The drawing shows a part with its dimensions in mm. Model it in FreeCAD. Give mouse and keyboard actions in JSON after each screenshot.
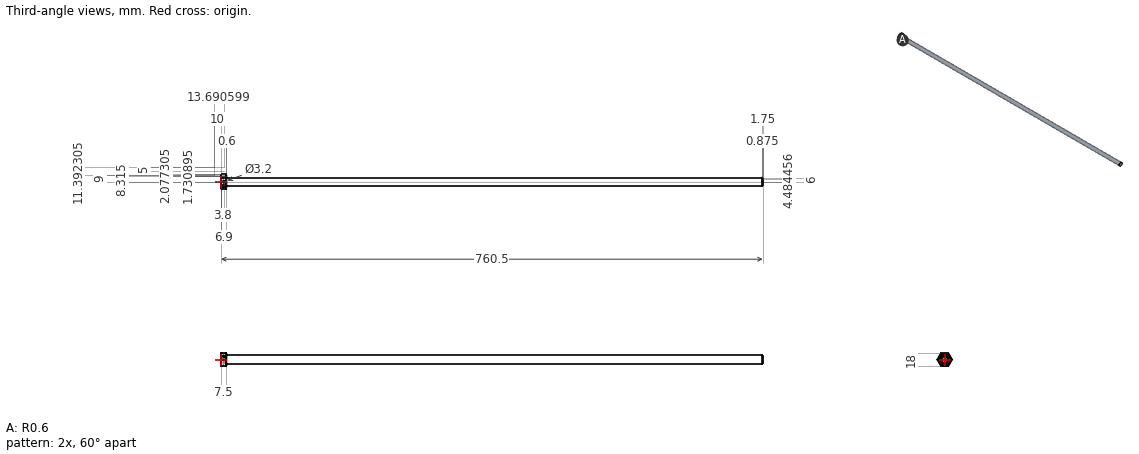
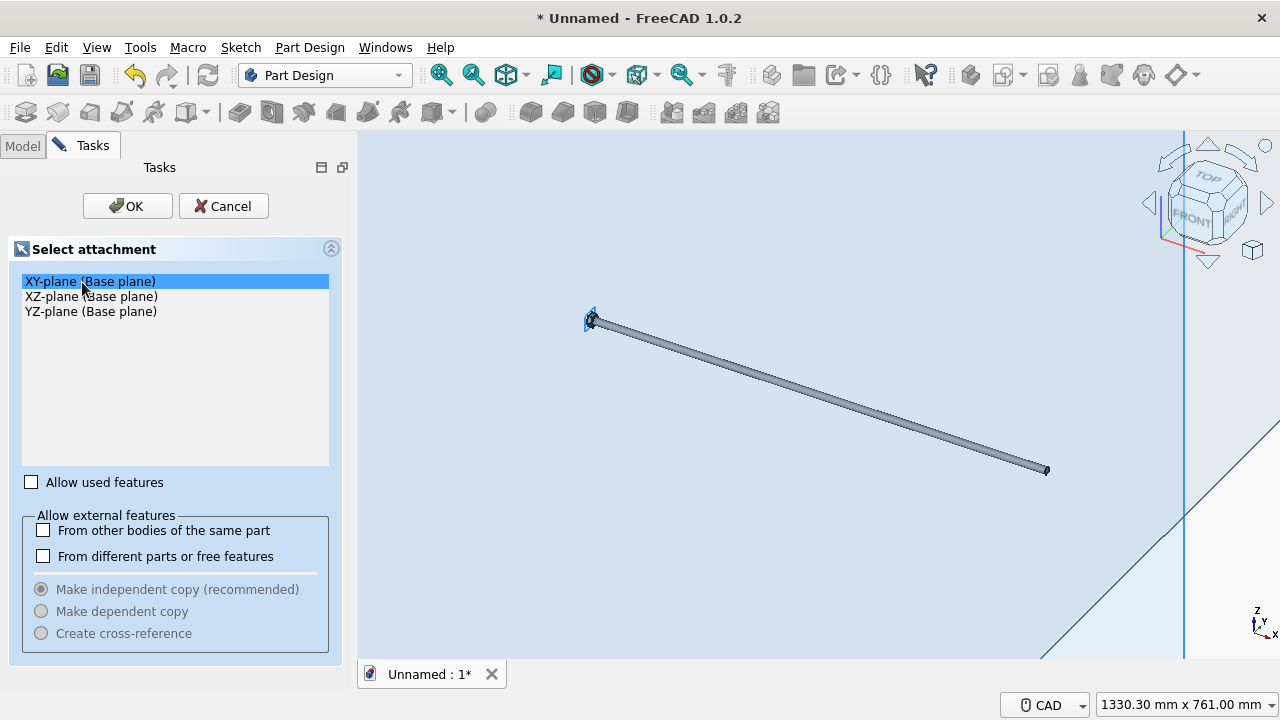
{"action": "left_click", "coordinate": [128, 206]}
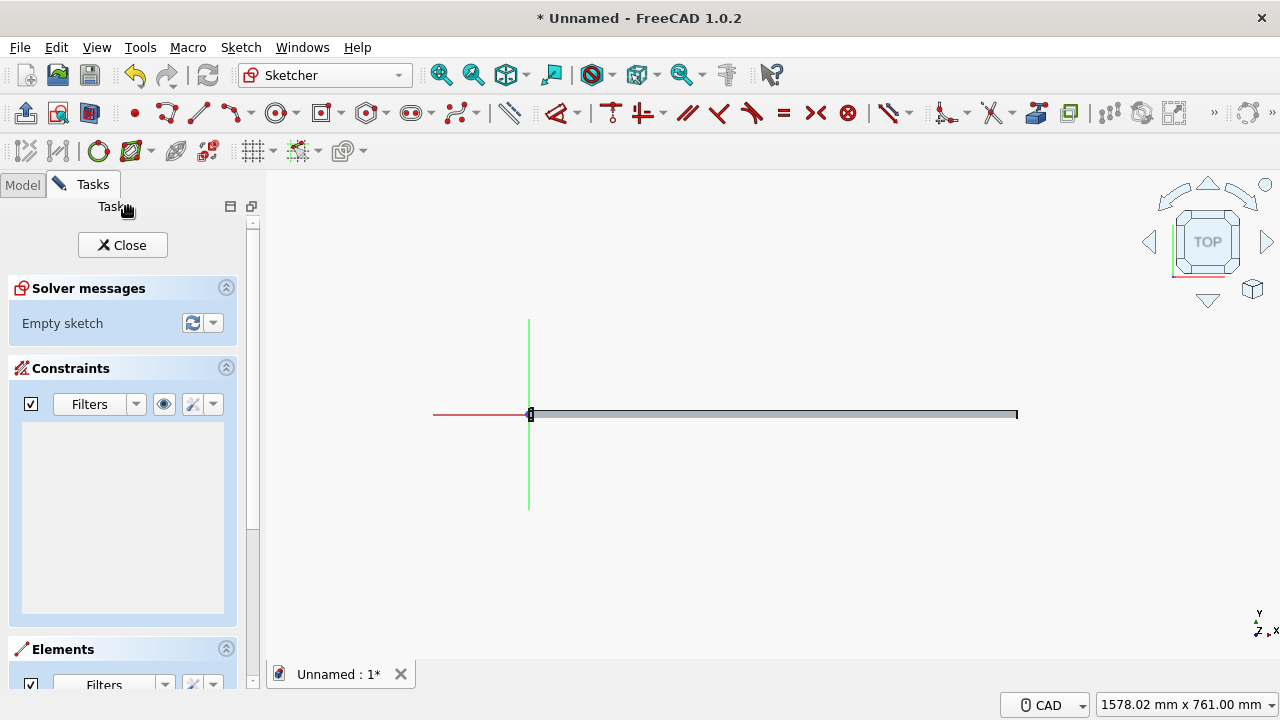
{"action": "key", "text": "q s"}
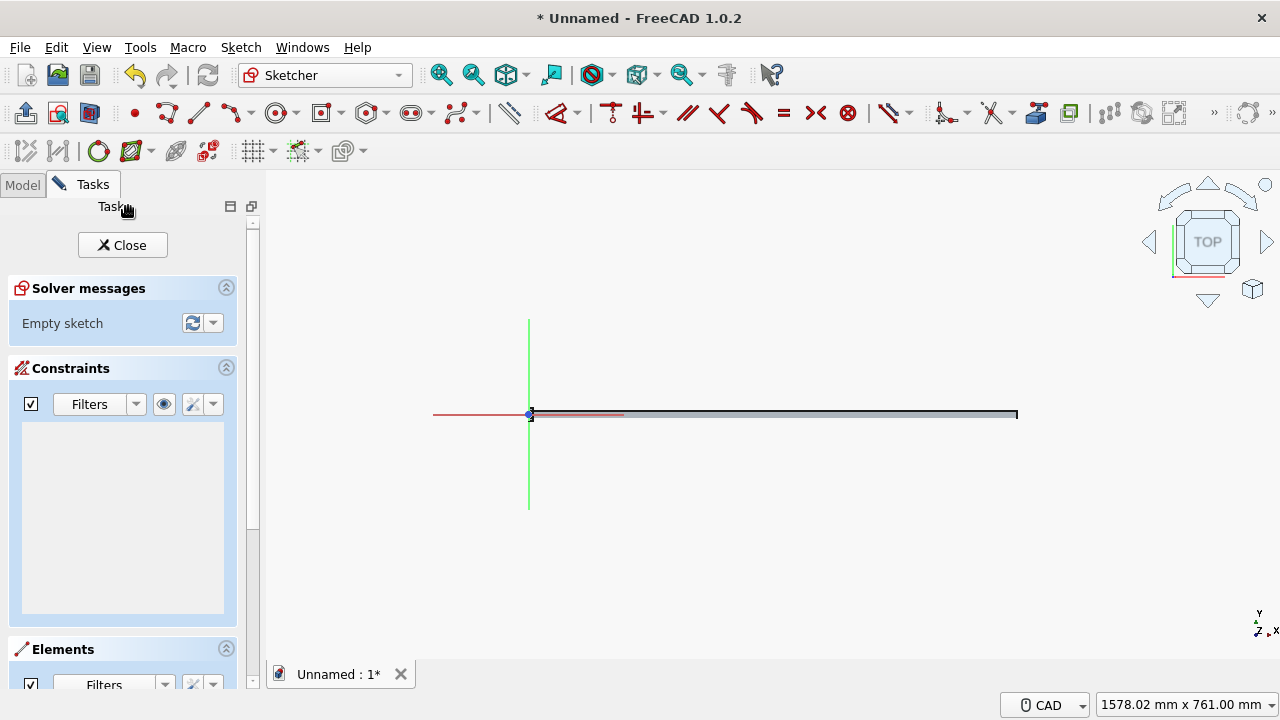
{"action": "scroll", "coordinate": [517, 408], "scroll_direction": "up", "scroll_amount": 15}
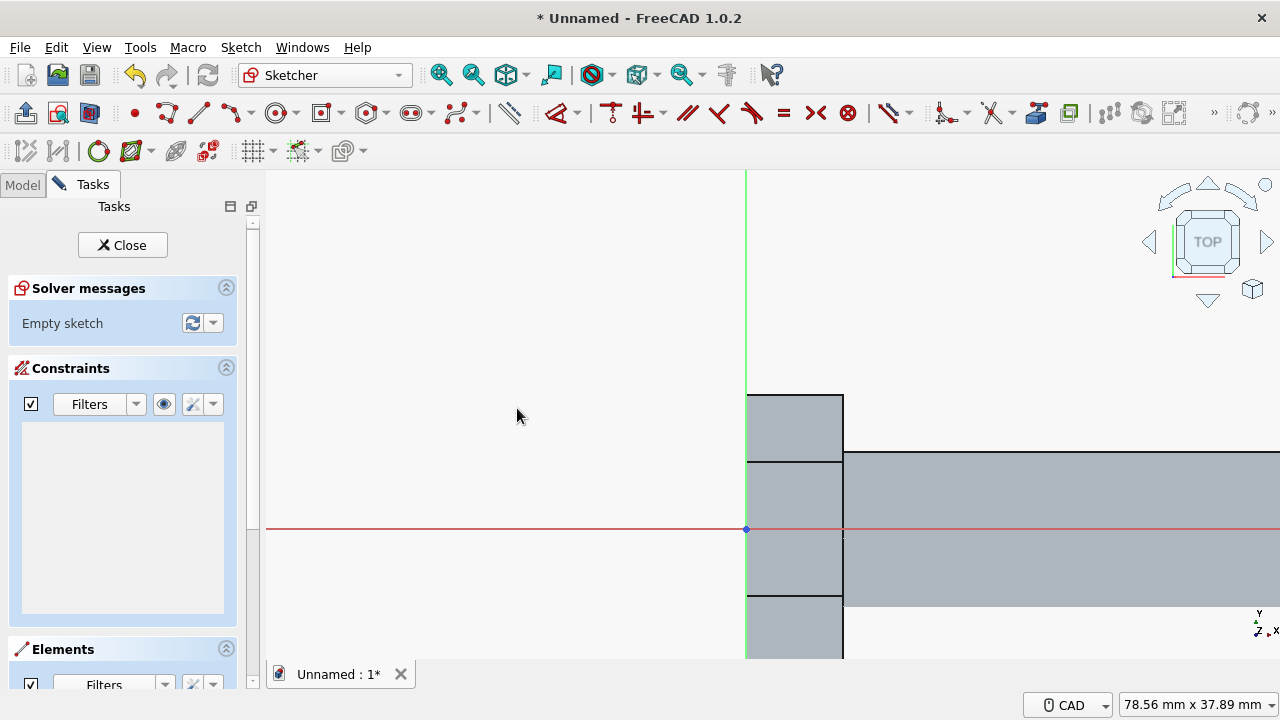
{"action": "key", "text": "g m"}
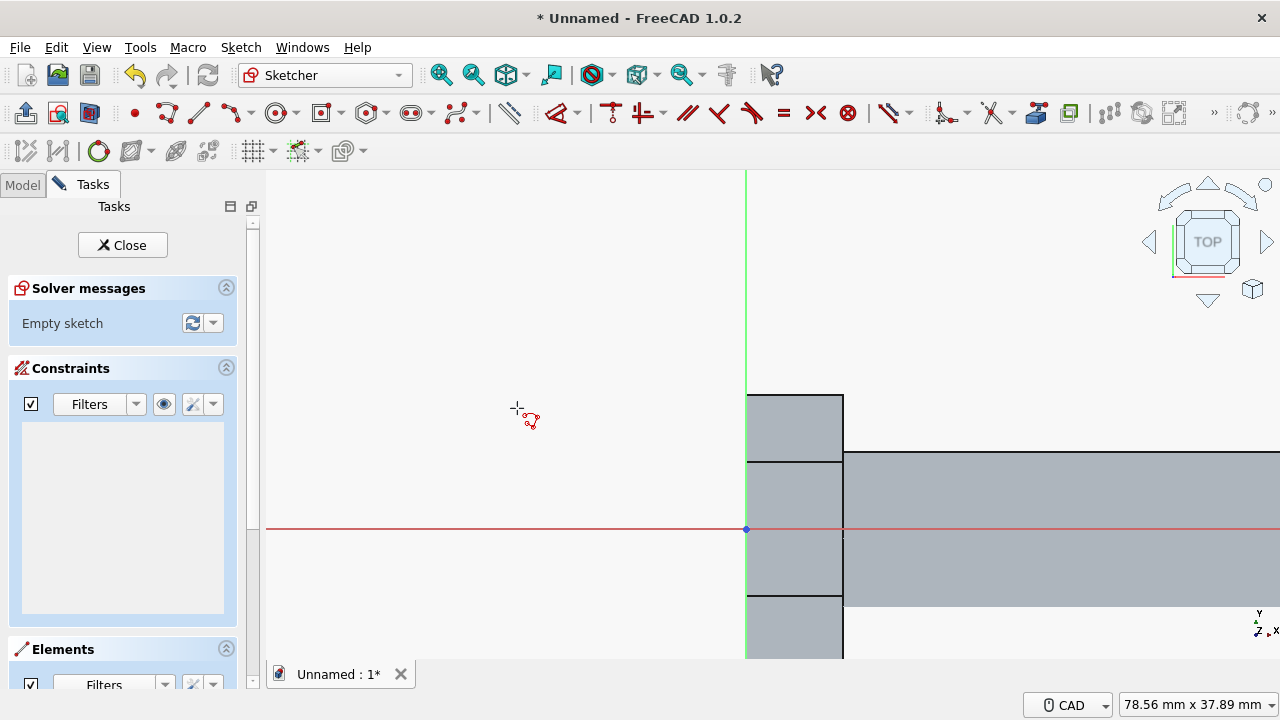
{"action": "left_click", "coordinate": [746, 413]}
{"action": "left_click", "coordinate": [794, 331]}
{"action": "left_click", "coordinate": [794, 266]}
{"action": "left_click", "coordinate": [617, 266]}
{"action": "left_click", "coordinate": [617, 413]}
{"action": "left_click", "coordinate": [746, 414]}
{"action": "key", "text": "Escape"}
{"action": "key", "text": "Escape"}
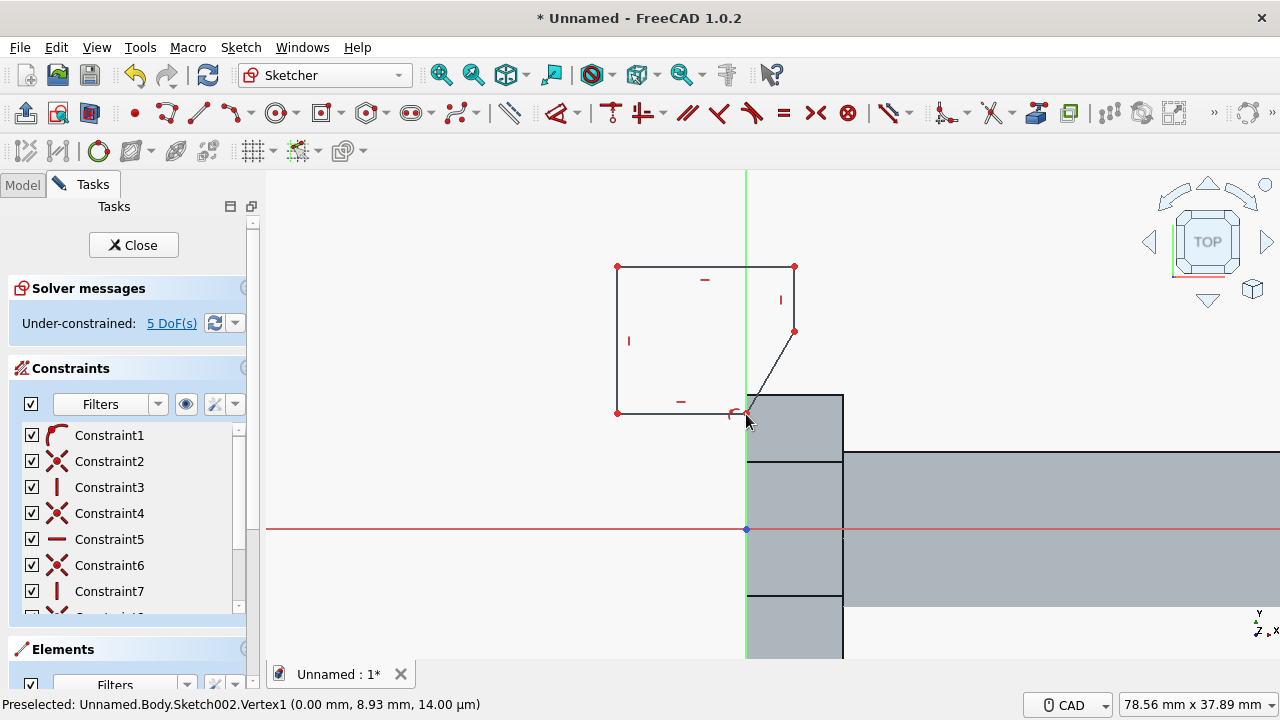
{"action": "key", "text": "d"}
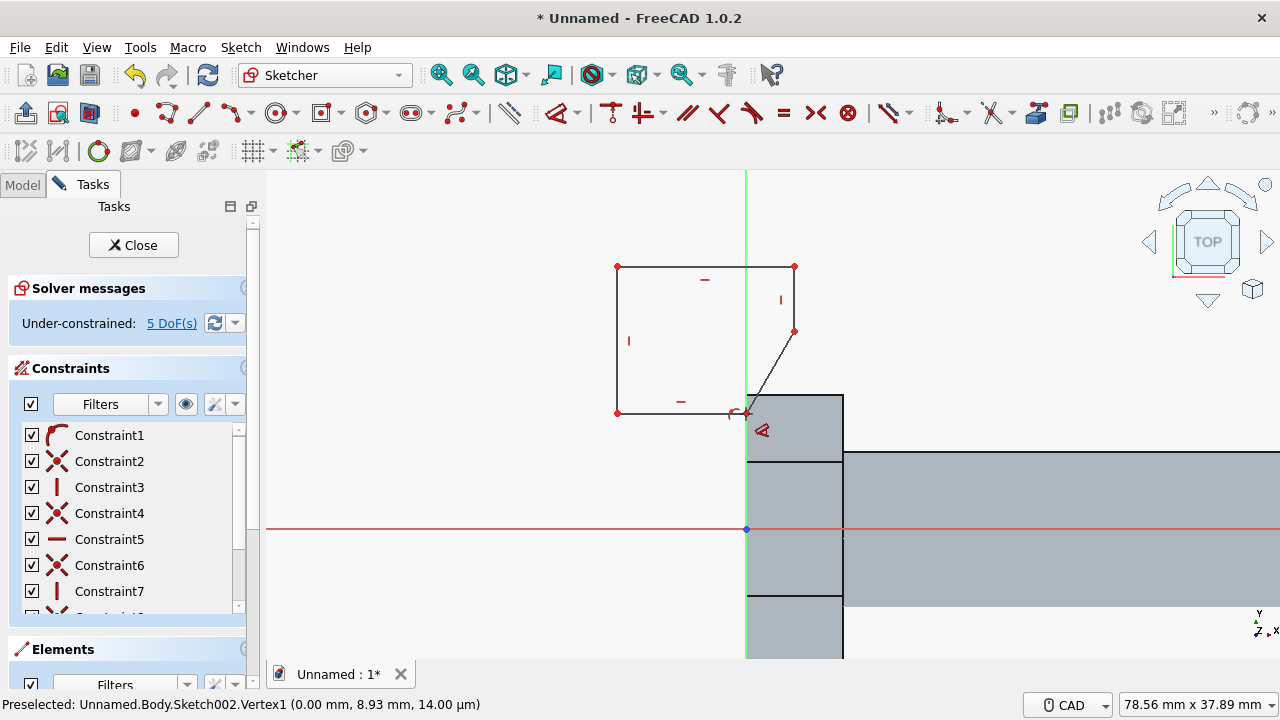
{"action": "left_click", "coordinate": [794, 313]}
{"action": "left_click", "coordinate": [828, 299]}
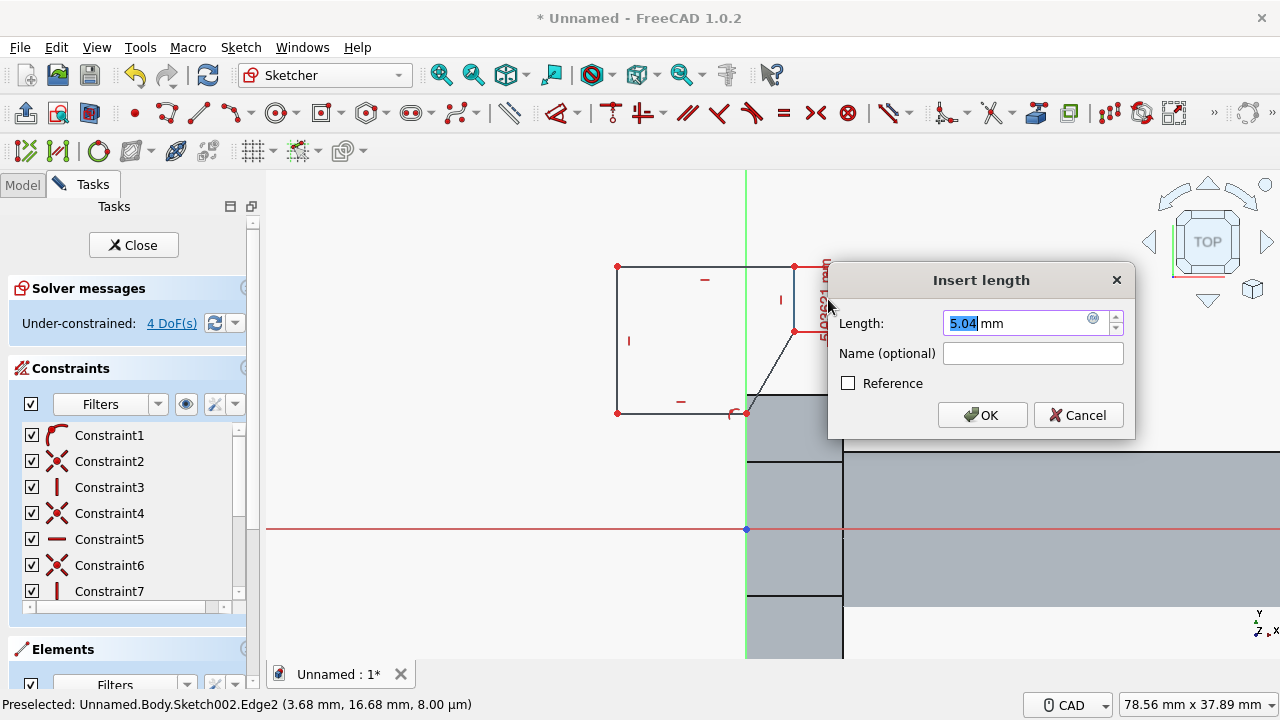
{"action": "type", "text": "5"}
{"action": "key", "text": "Return"}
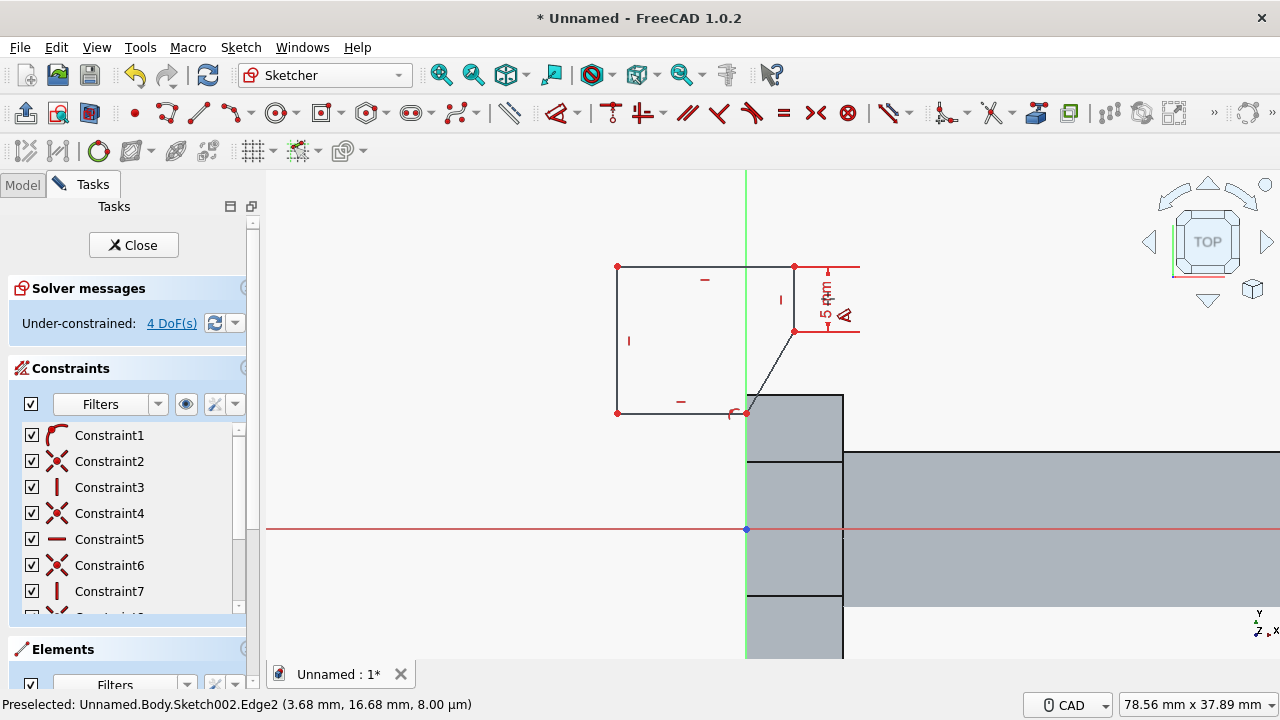
{"action": "left_click", "coordinate": [656, 414]}
{"action": "left_click", "coordinate": [682, 448]}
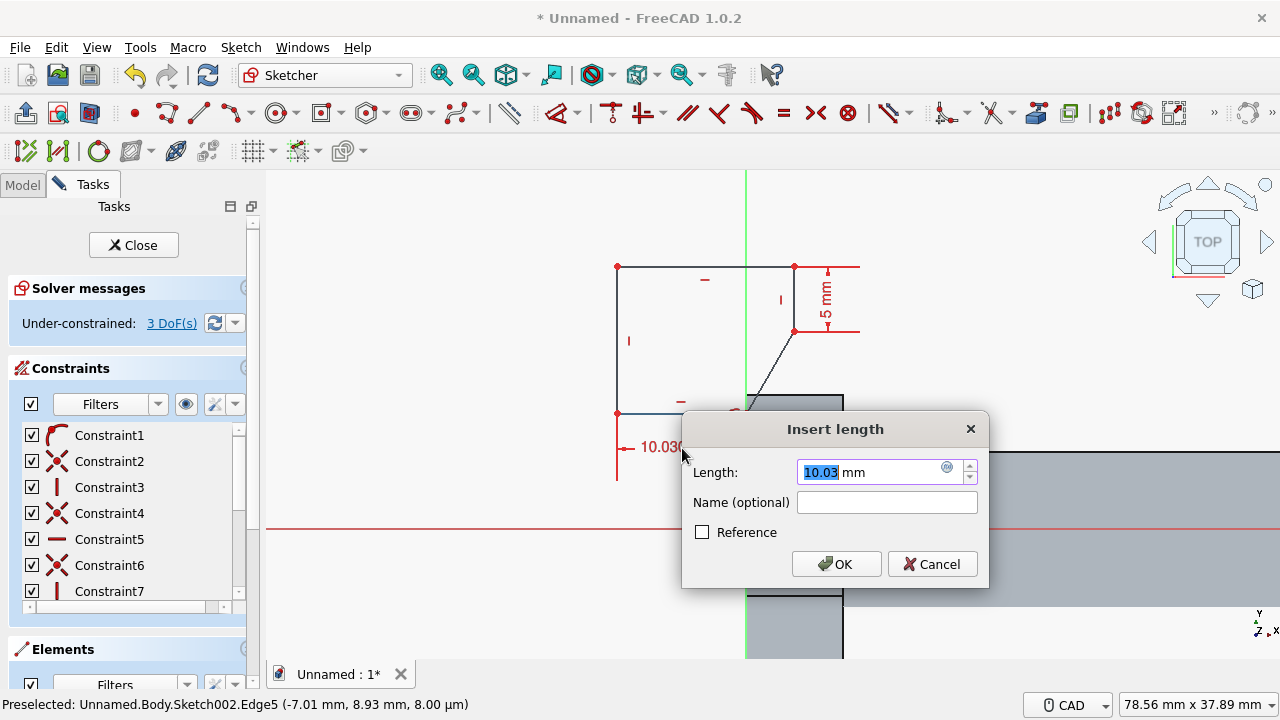
{"action": "type", "text": "10"}
{"action": "key", "text": "Return"}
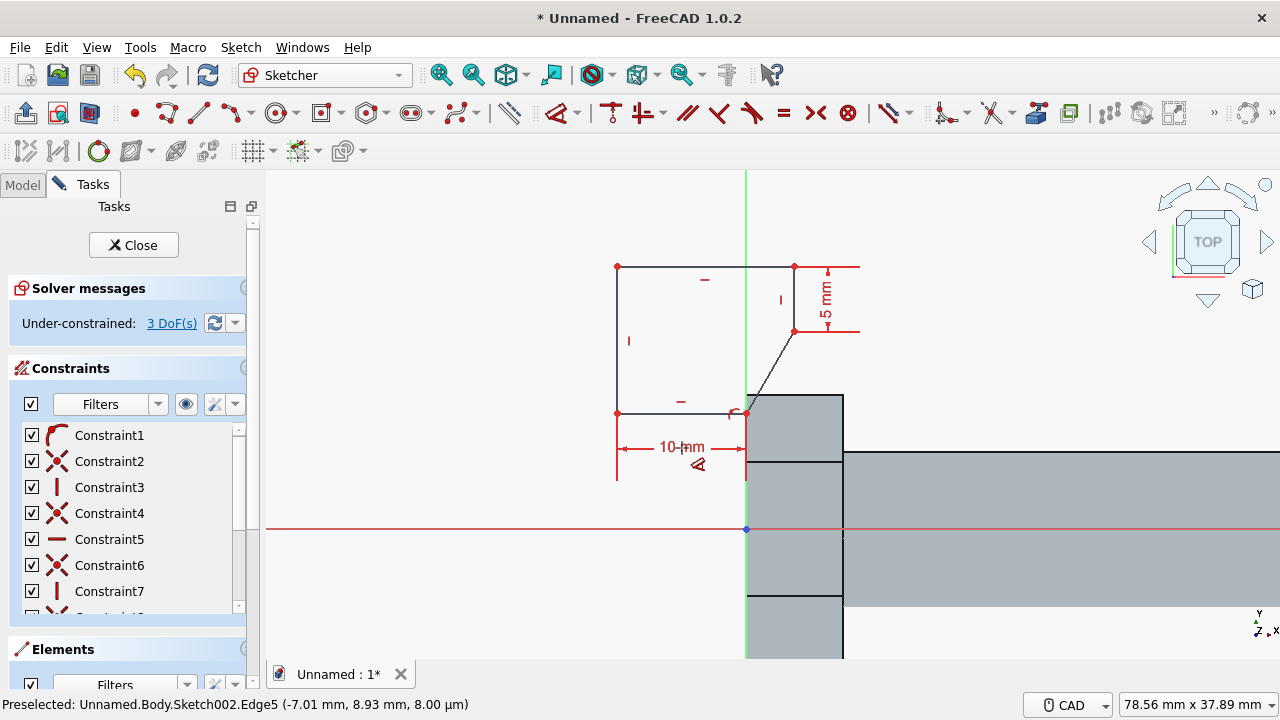
{"action": "left_click", "coordinate": [746, 414]}
{"action": "left_click", "coordinate": [780, 472]}